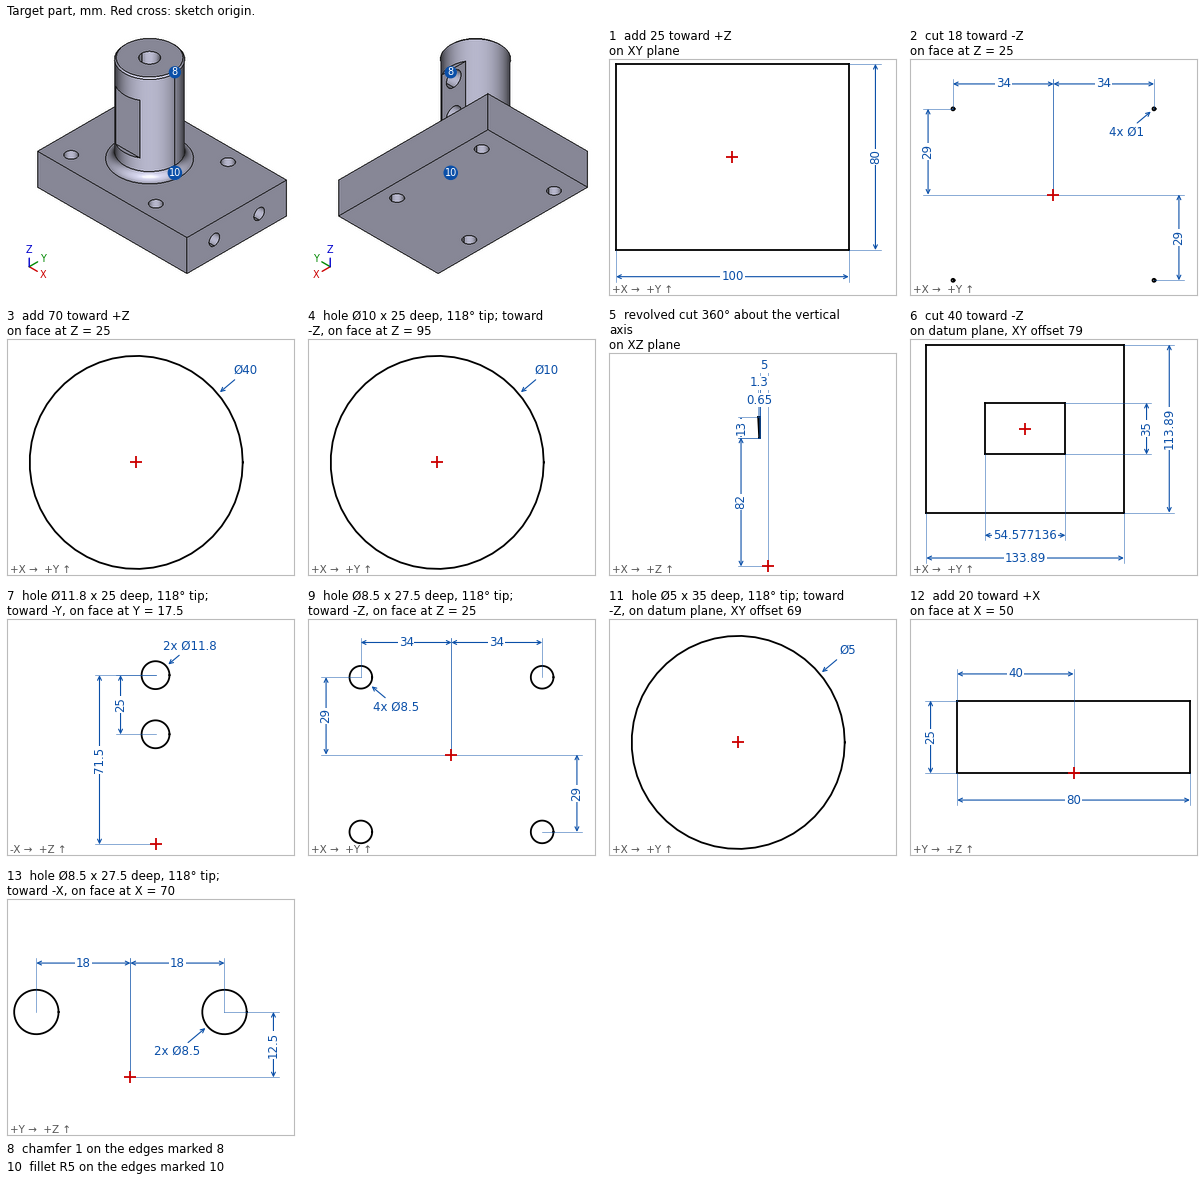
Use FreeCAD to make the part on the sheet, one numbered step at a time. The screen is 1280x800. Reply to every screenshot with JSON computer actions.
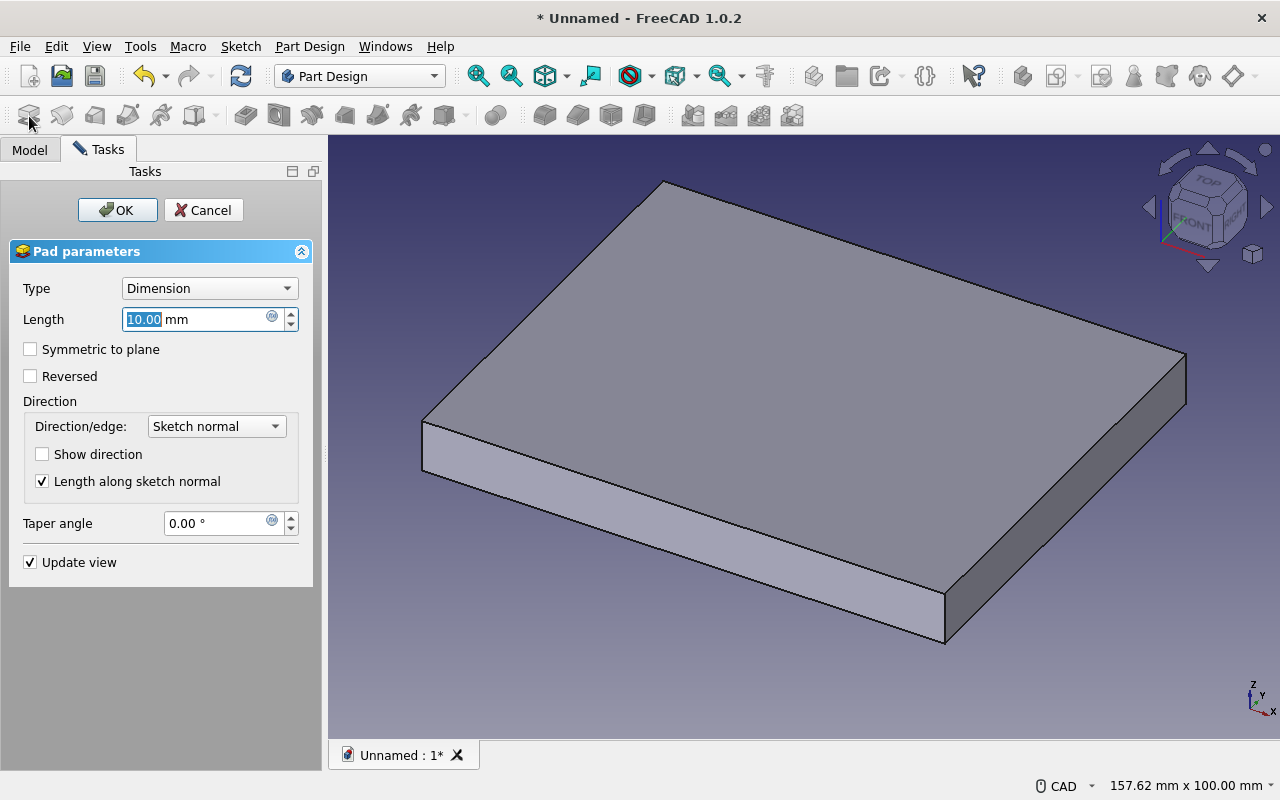
{"action": "type", "text": "25"}
{"action": "key", "text": "Tab"}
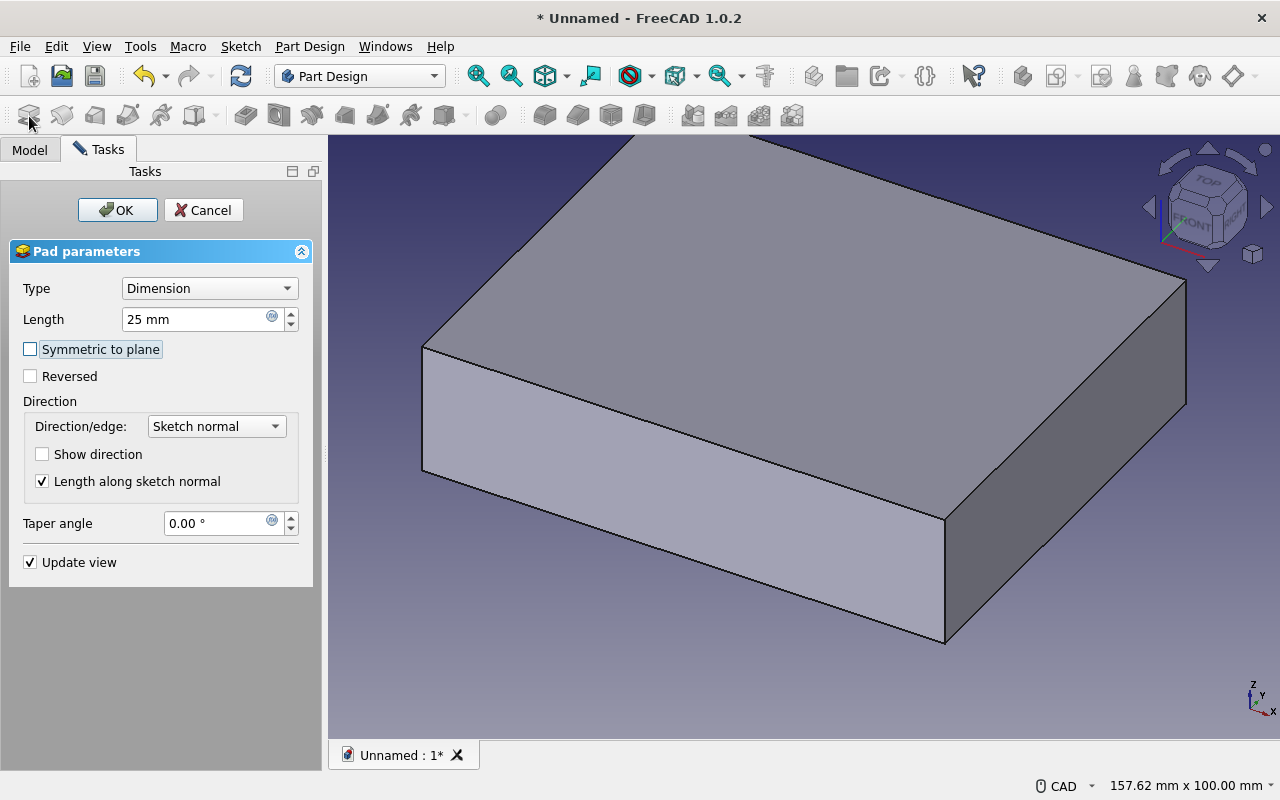
{"action": "left_click", "coordinate": [118, 210]}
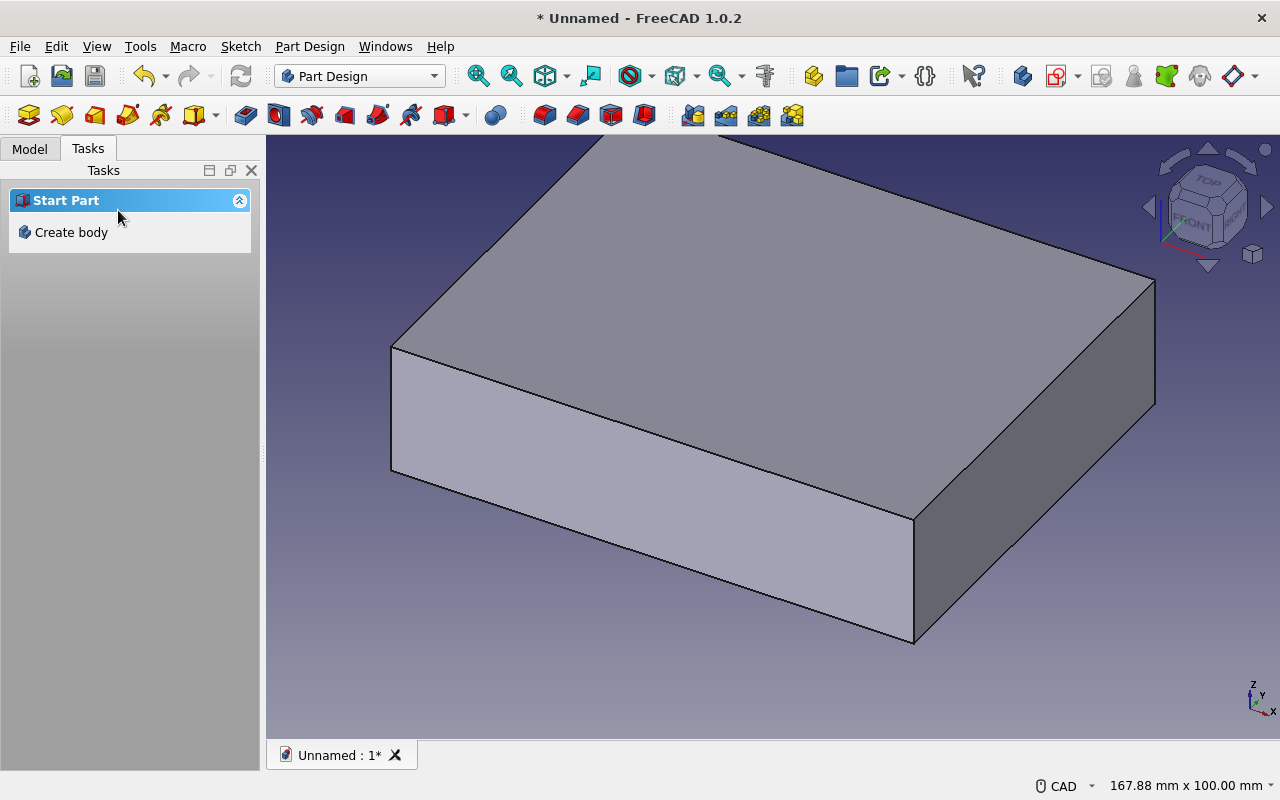
{"action": "left_click", "coordinate": [479, 76]}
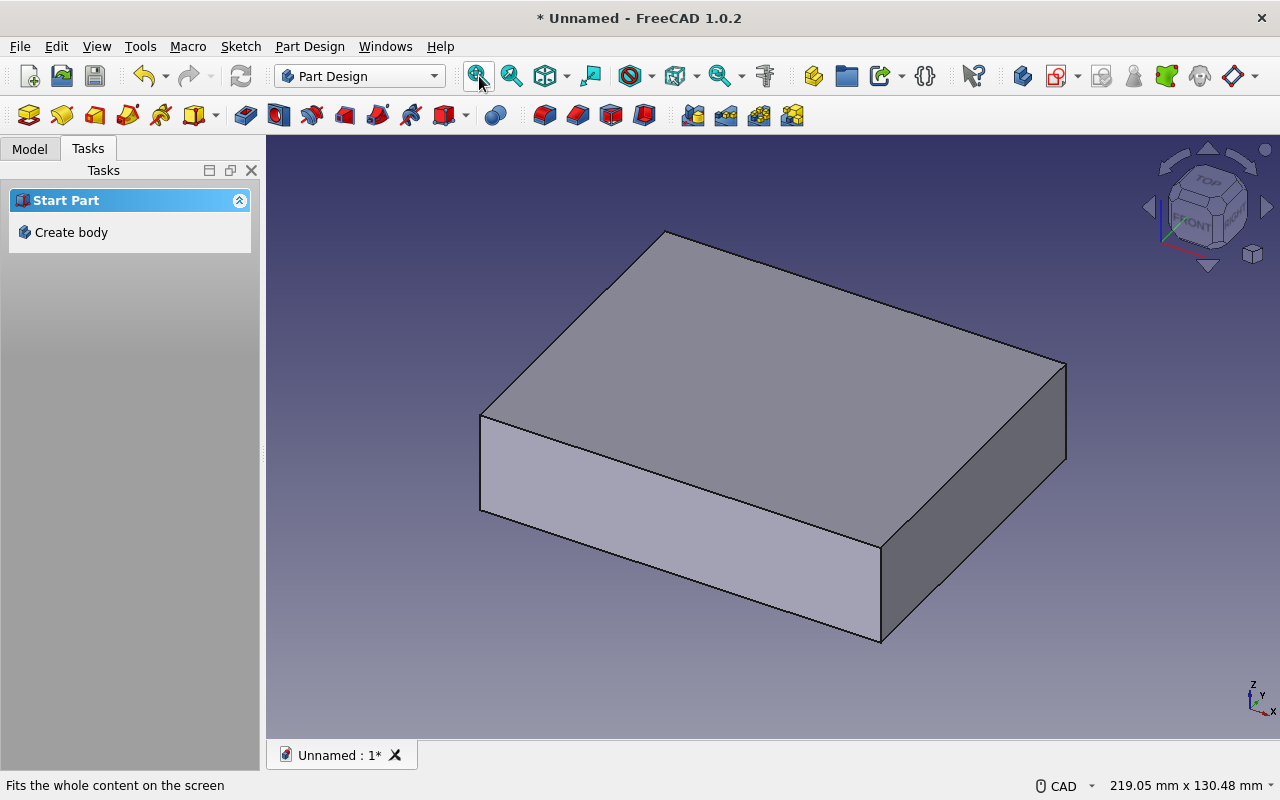
{"action": "left_click", "coordinate": [773, 389]}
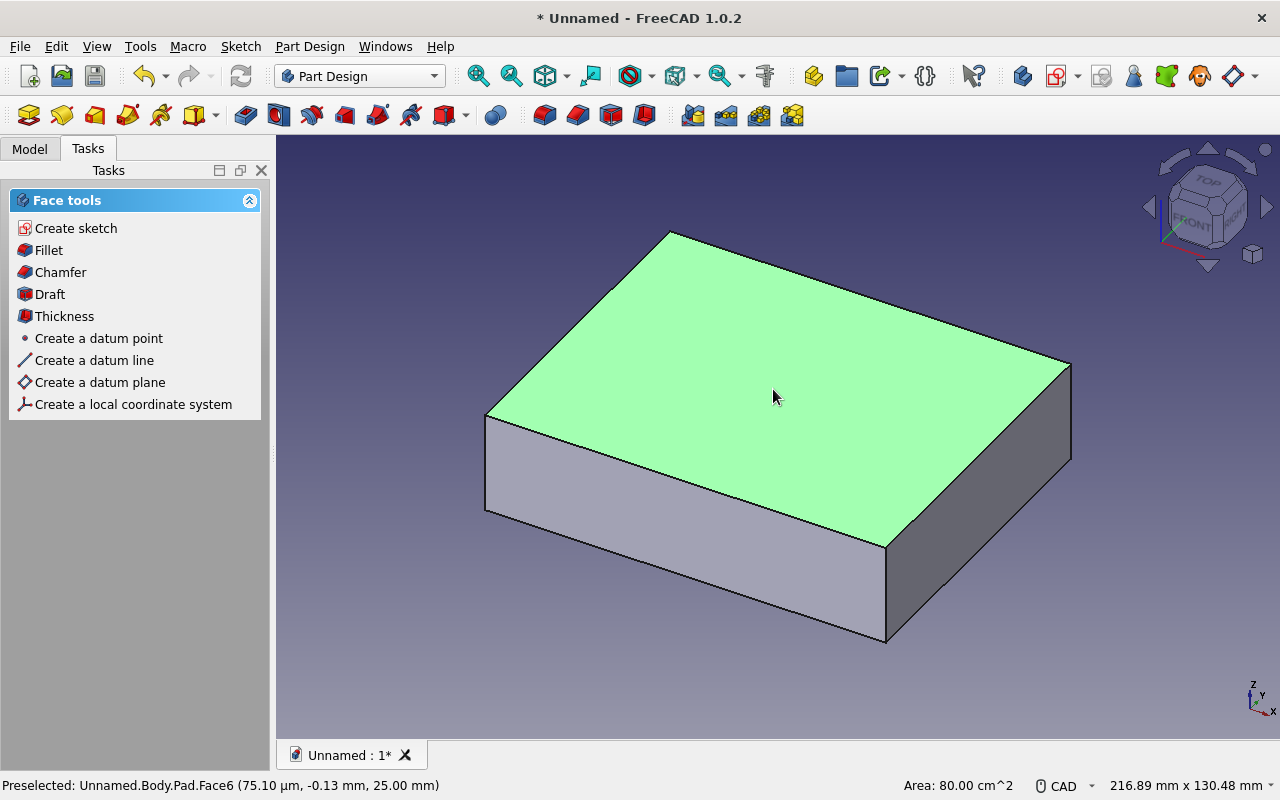
{"action": "left_click", "coordinate": [1056, 76]}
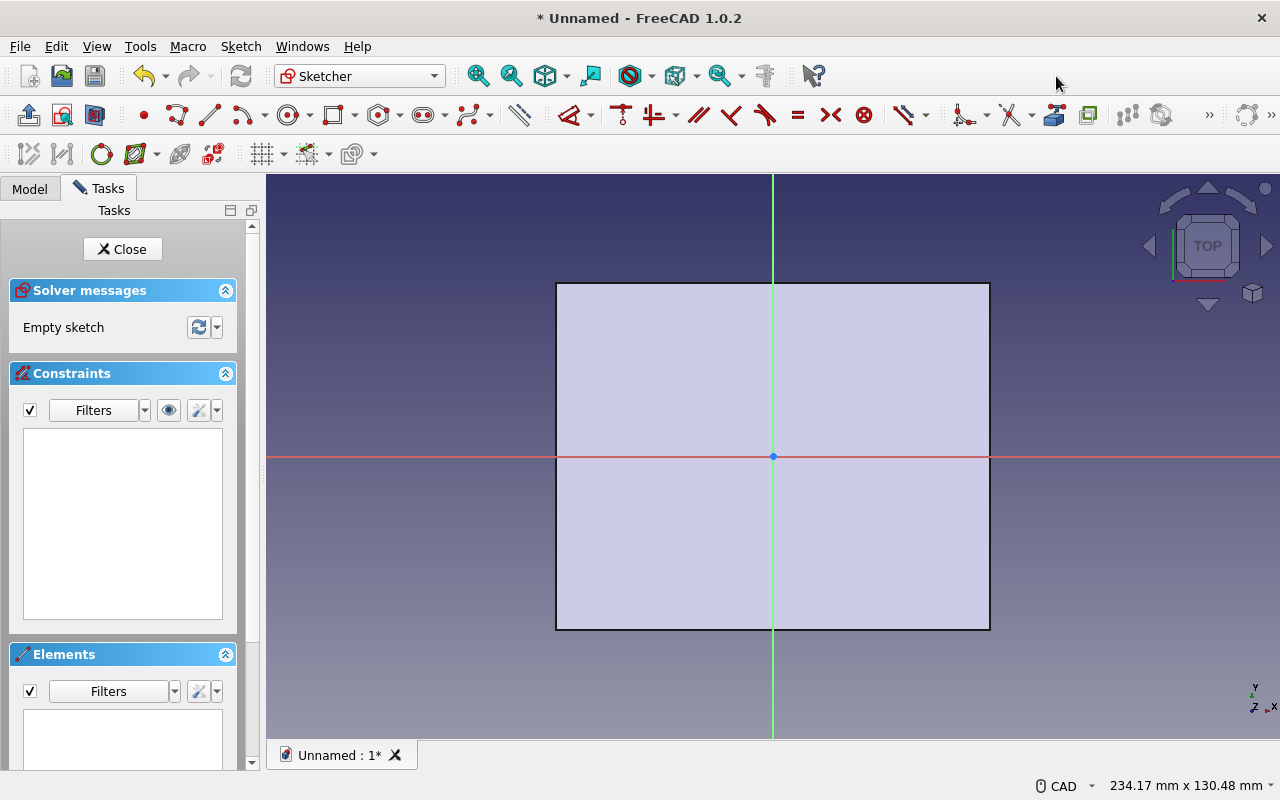
{"action": "scroll", "coordinate": [912, 456], "scroll_direction": "up", "scroll_amount": 2}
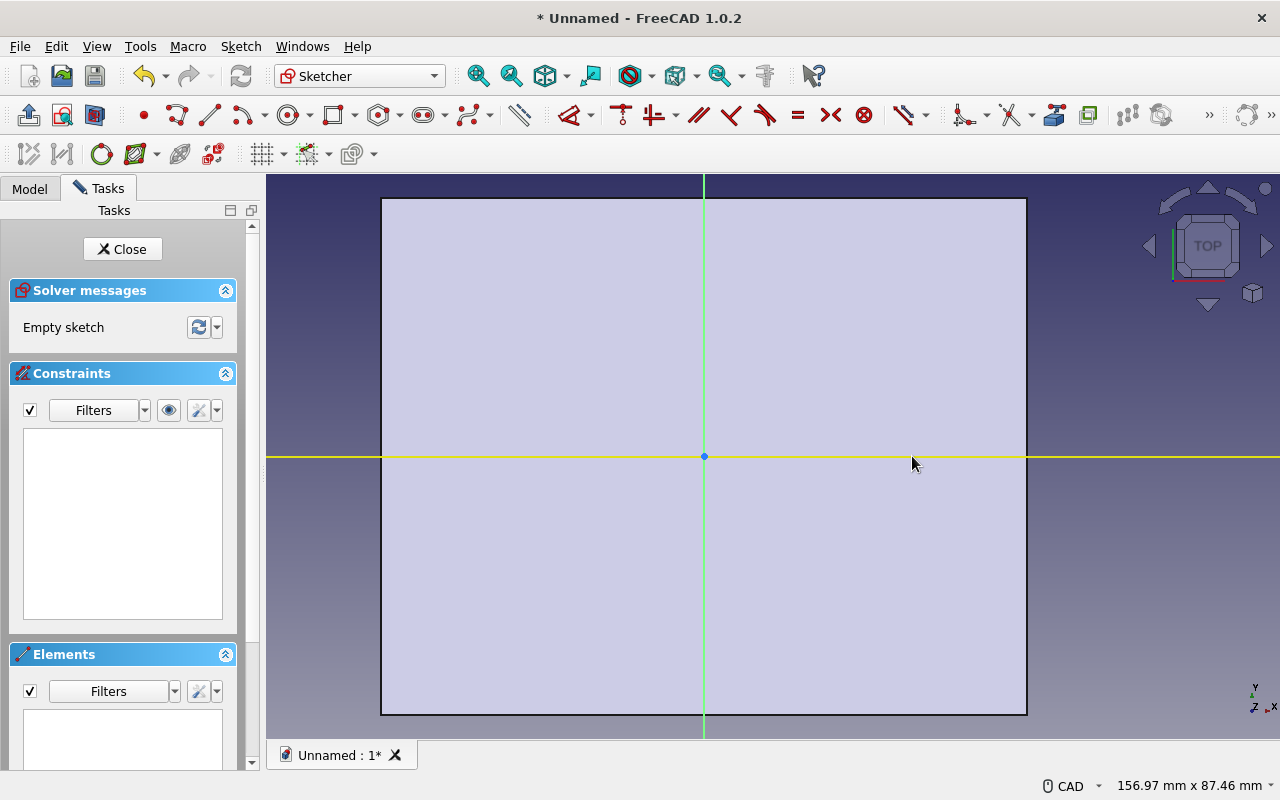
{"action": "key", "text": "g c"}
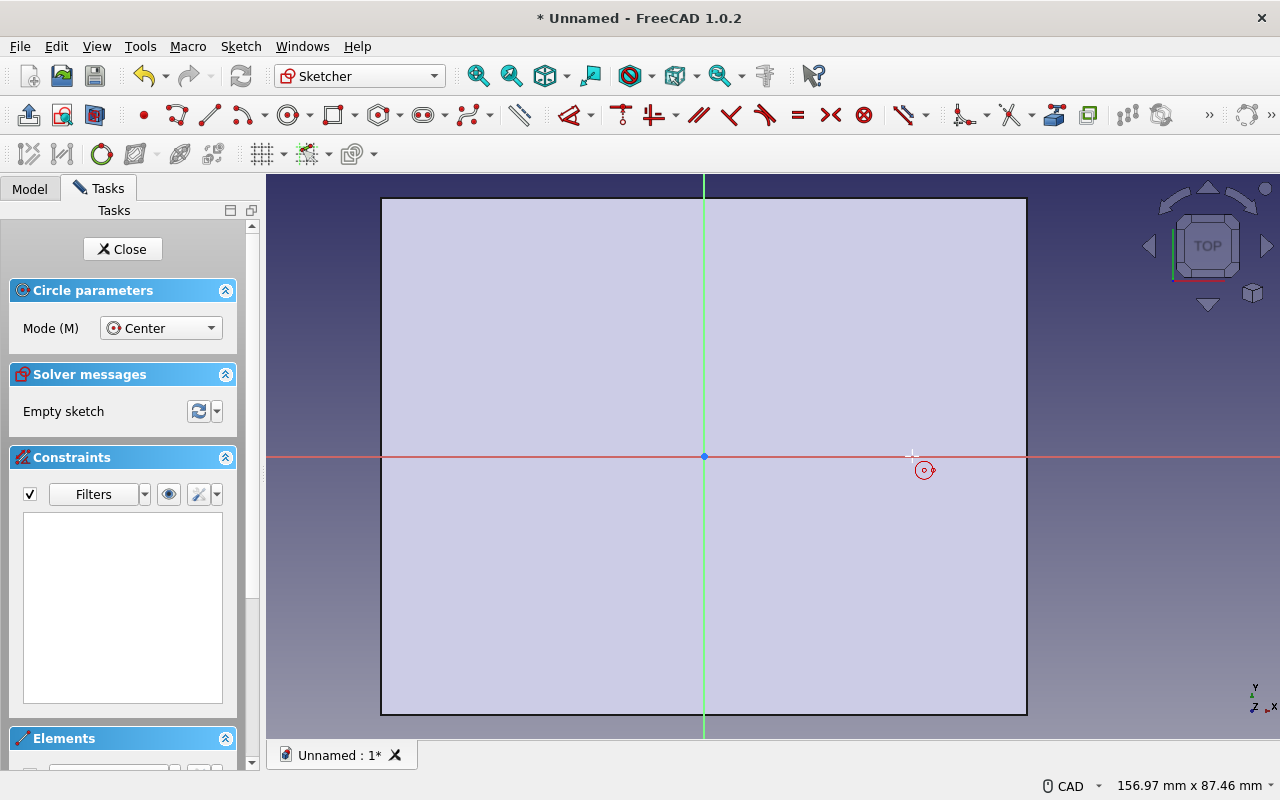
{"action": "scroll", "coordinate": [485, 269], "scroll_direction": "up", "scroll_amount": 10}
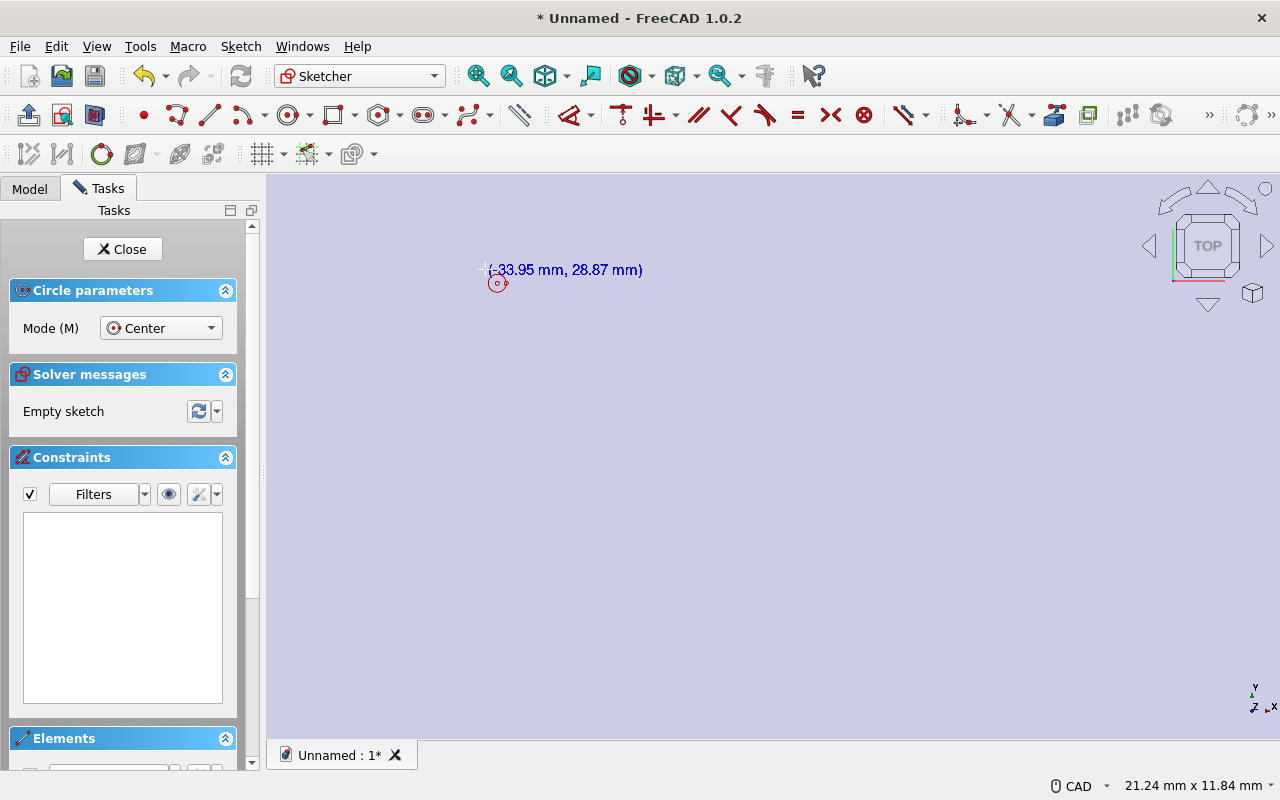
{"action": "scroll", "coordinate": [485, 269], "scroll_direction": "down", "scroll_amount": 10}